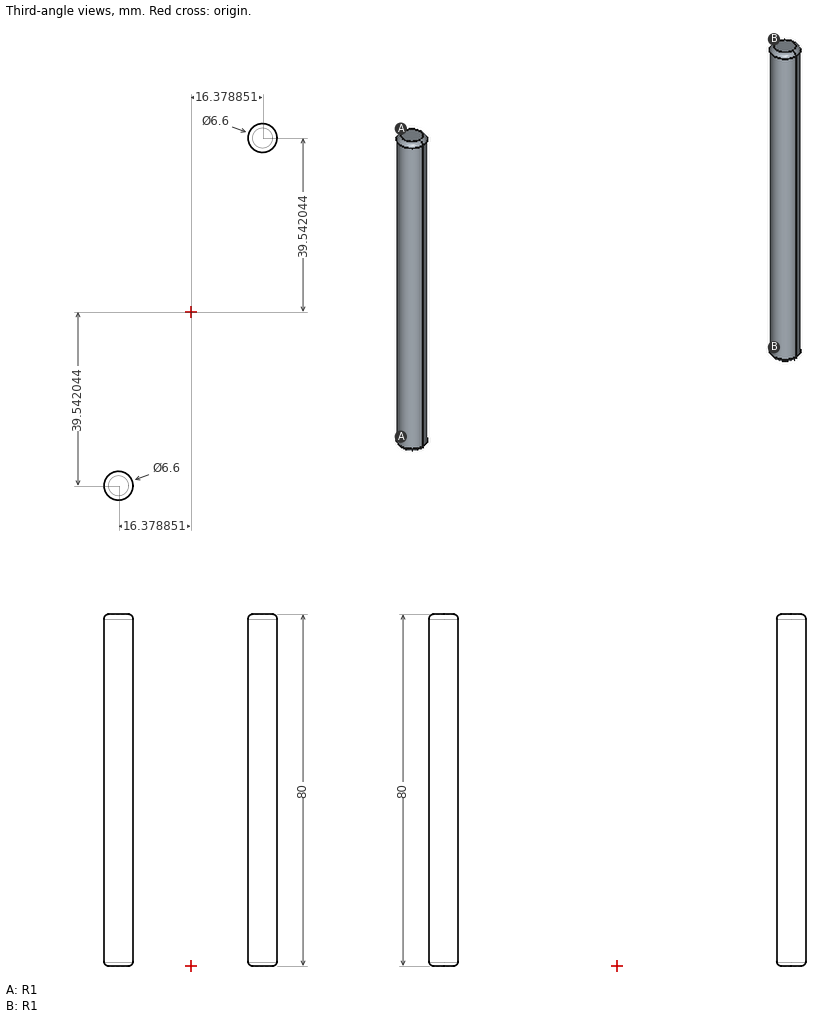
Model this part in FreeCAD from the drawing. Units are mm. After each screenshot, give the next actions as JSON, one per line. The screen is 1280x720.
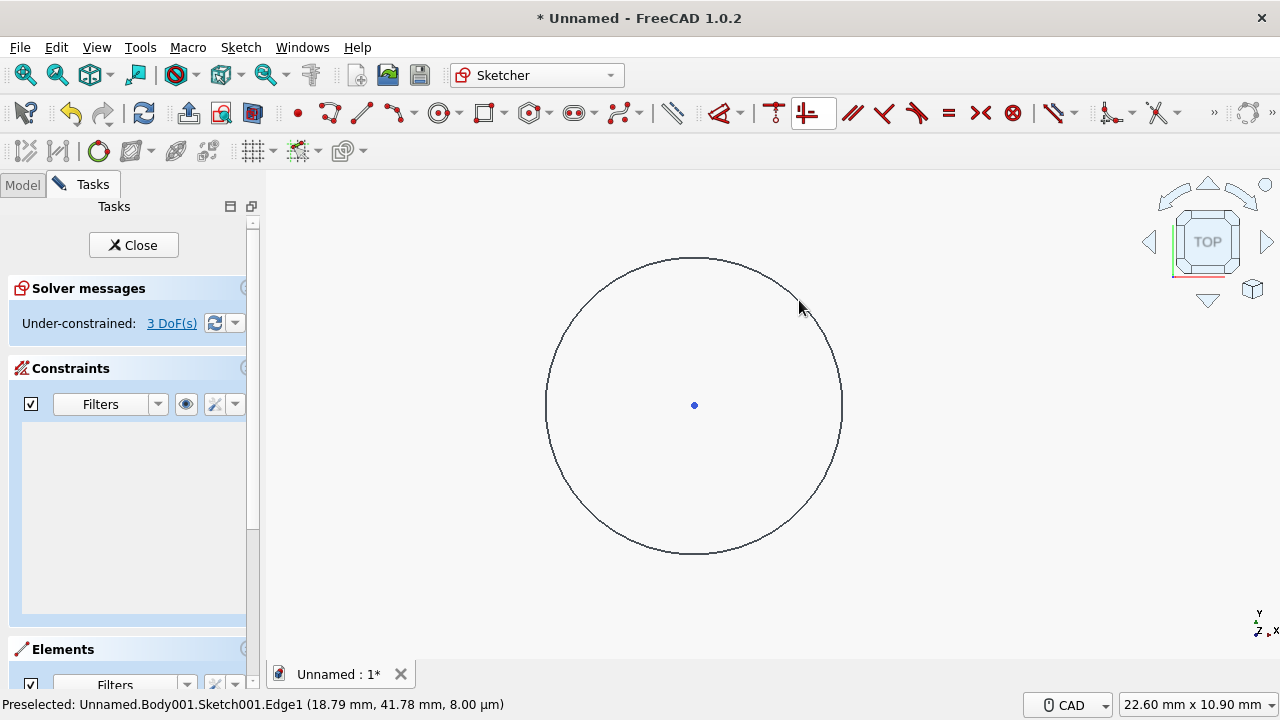
{"action": "left_click", "coordinate": [720, 114]}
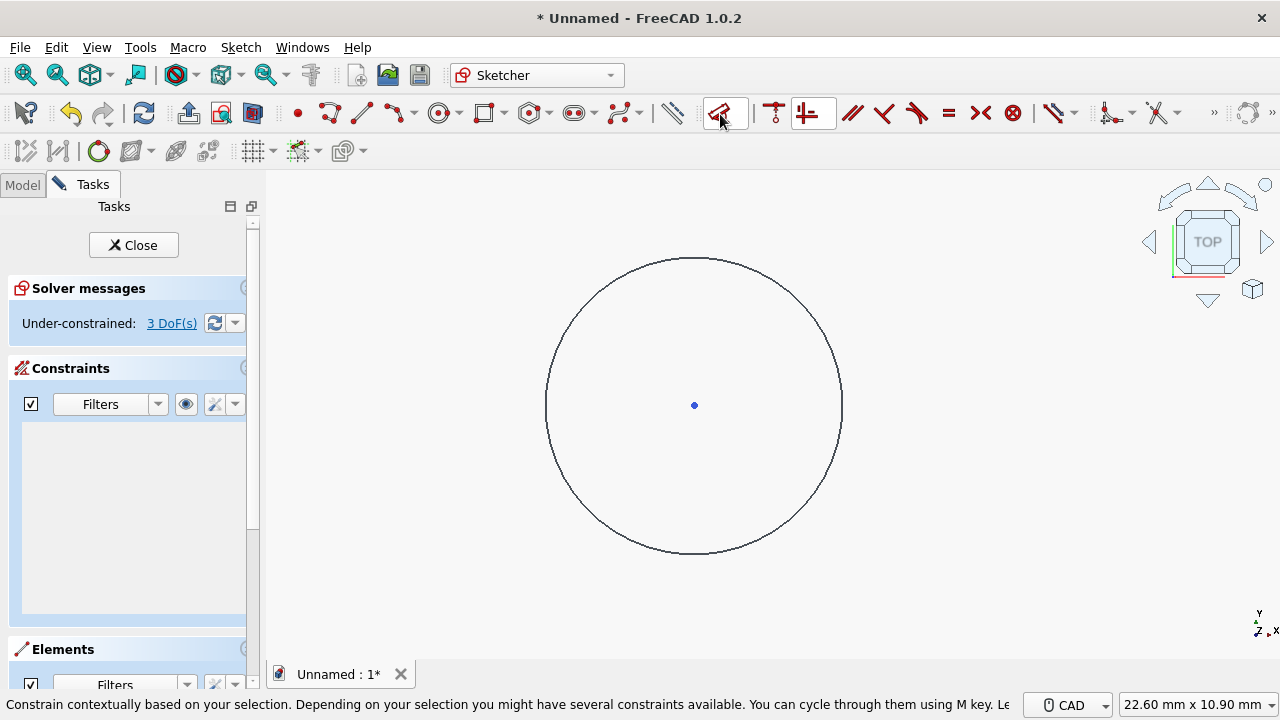
{"action": "left_click", "coordinate": [799, 301]}
{"action": "left_click", "coordinate": [822, 278]}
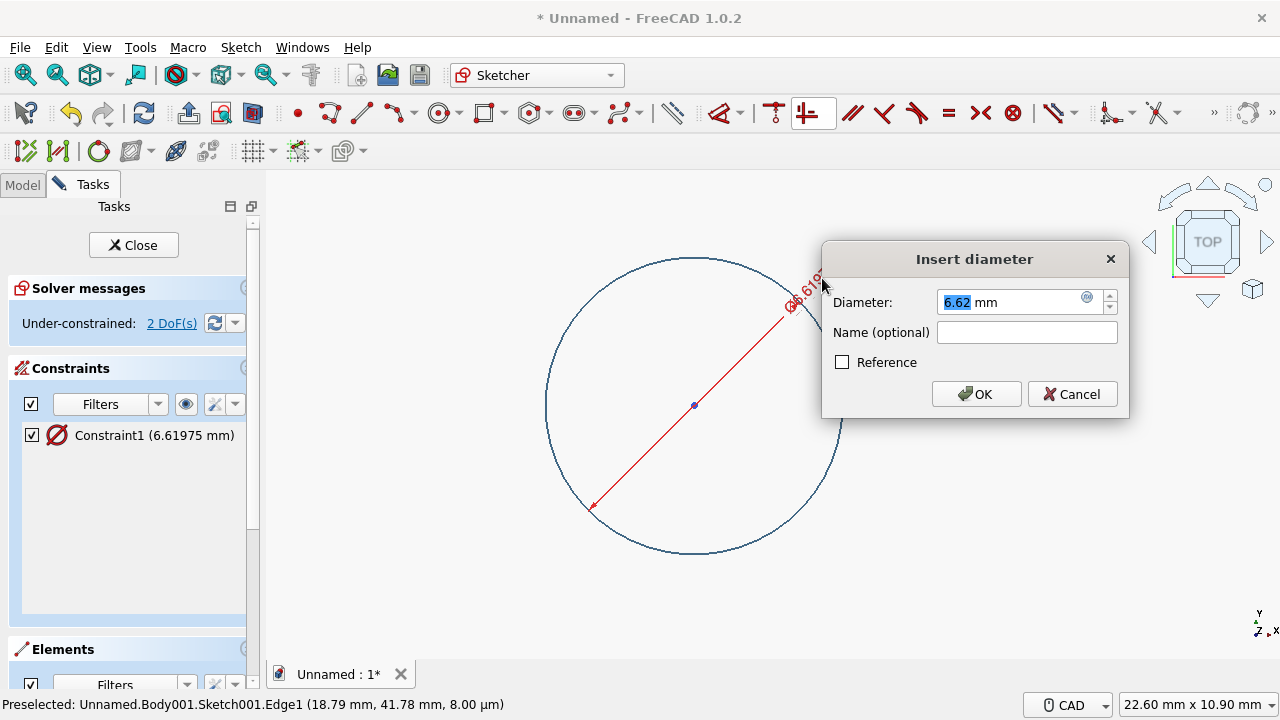
{"action": "type", "text": "6.6"}
{"action": "key", "text": "Return"}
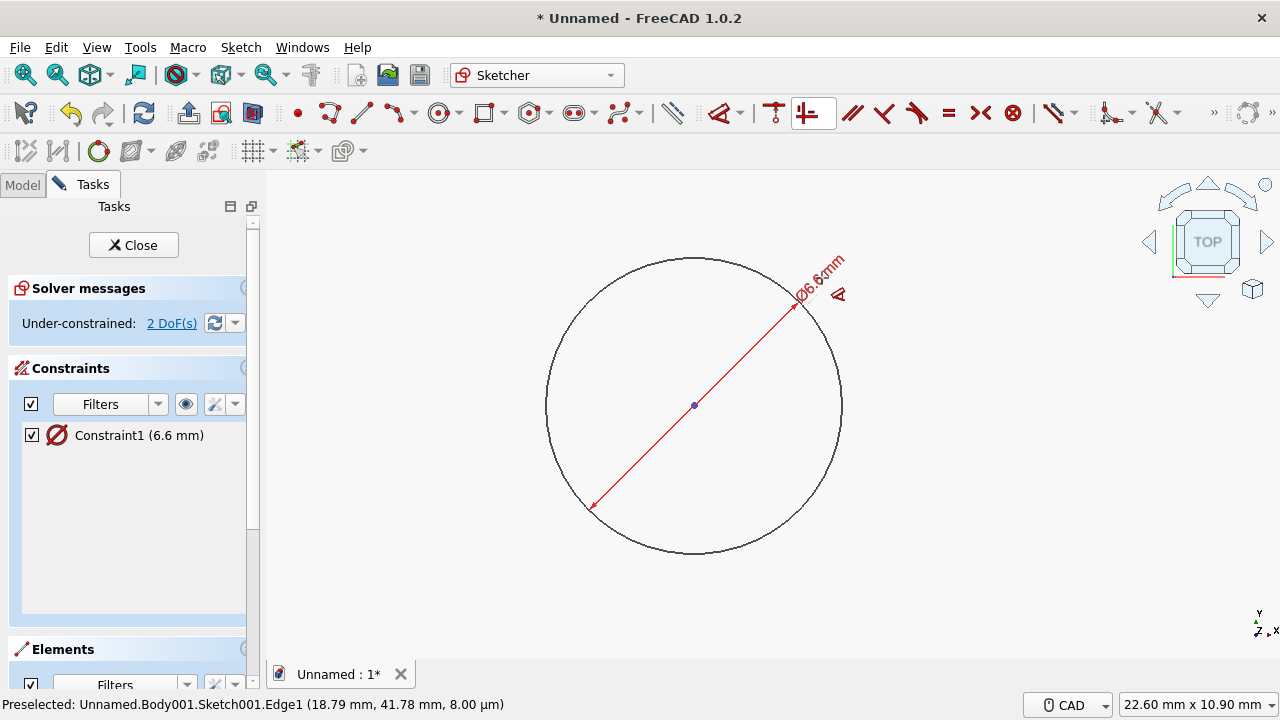
{"action": "left_click", "coordinate": [694, 406]}
{"action": "left_click", "coordinate": [494, 372]}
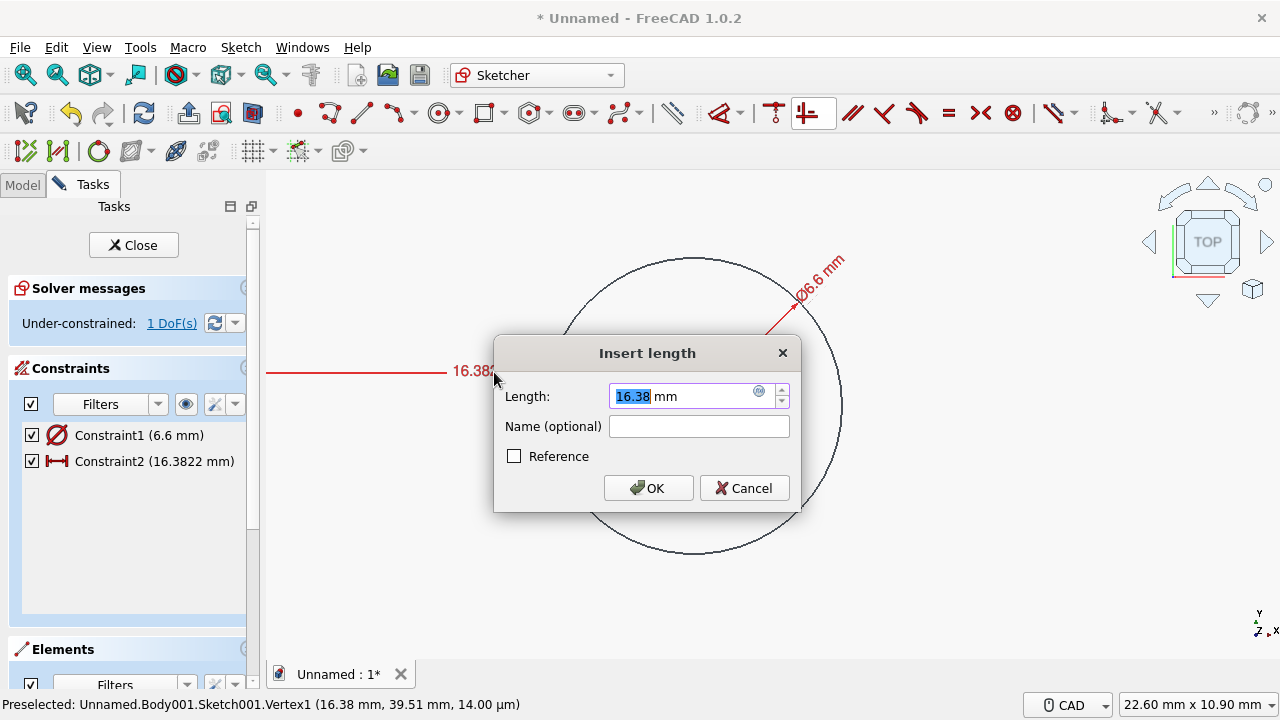
{"action": "type", "text": "16.378851"}
{"action": "key", "text": "Return"}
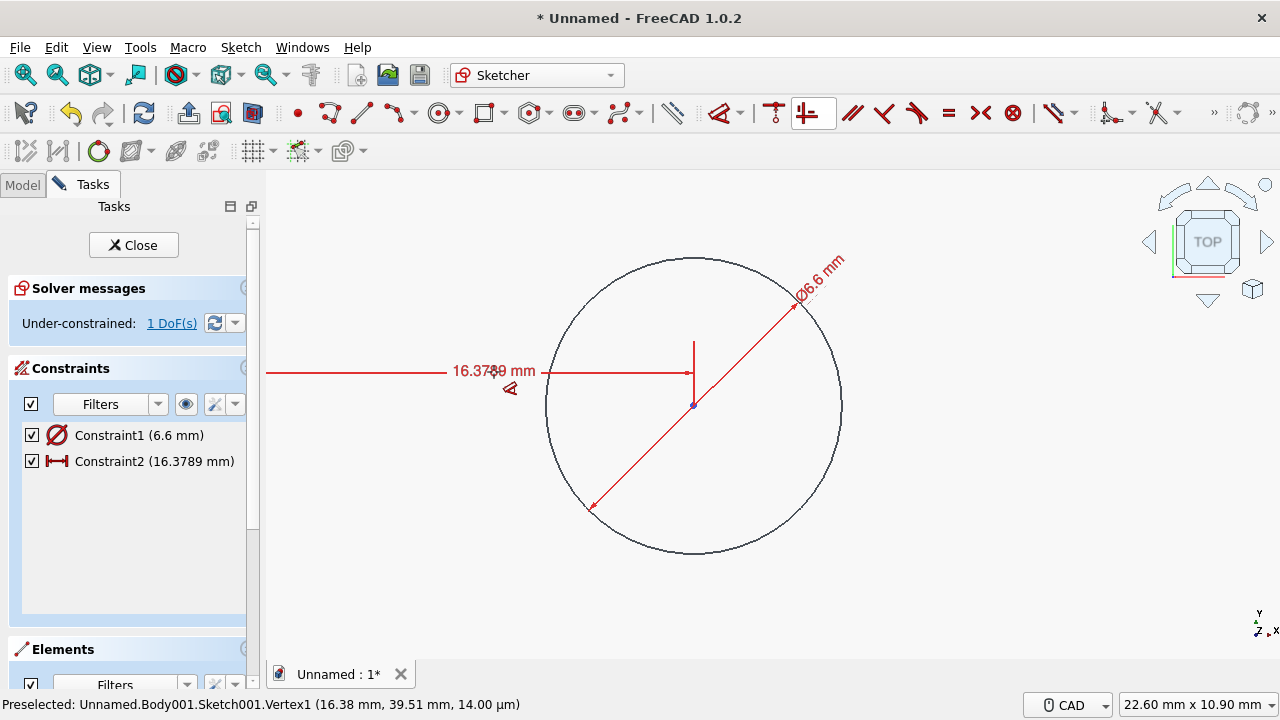
{"action": "left_click", "coordinate": [694, 406]}
{"action": "left_click", "coordinate": [728, 518]}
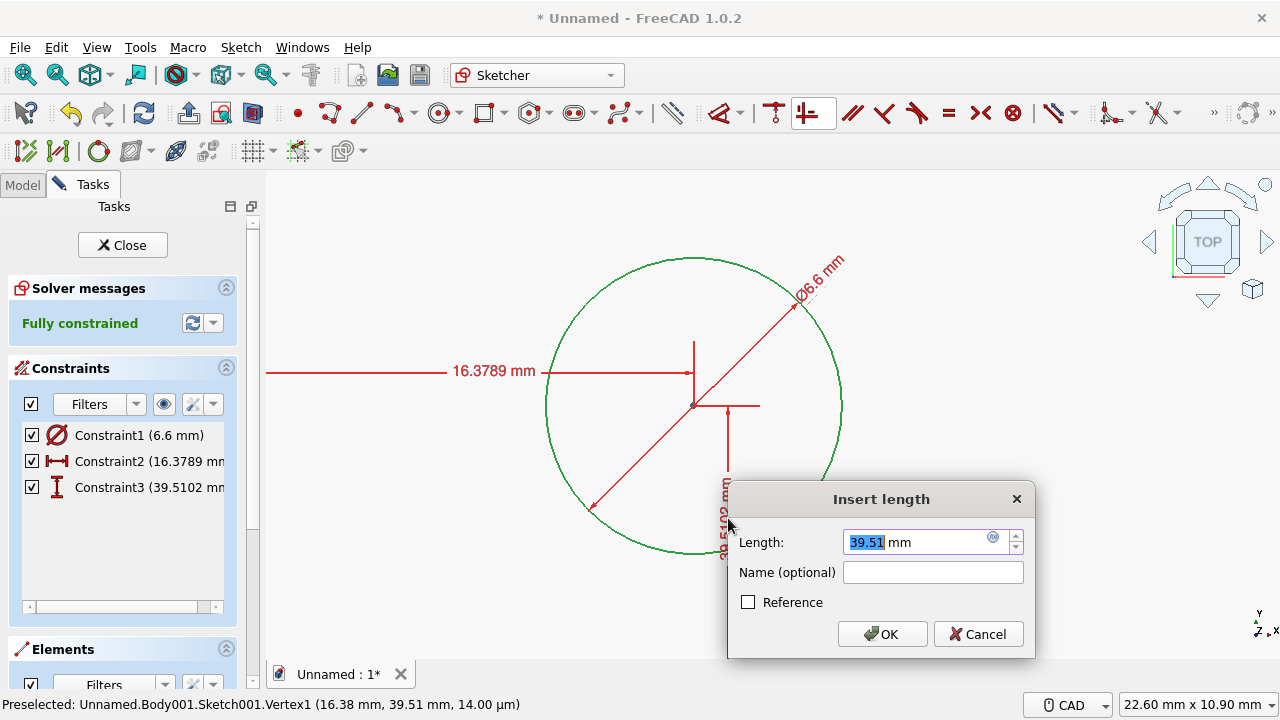
{"action": "type", "text": "39.542044"}
{"action": "key", "text": "Return"}
{"action": "key", "text": "Escape"}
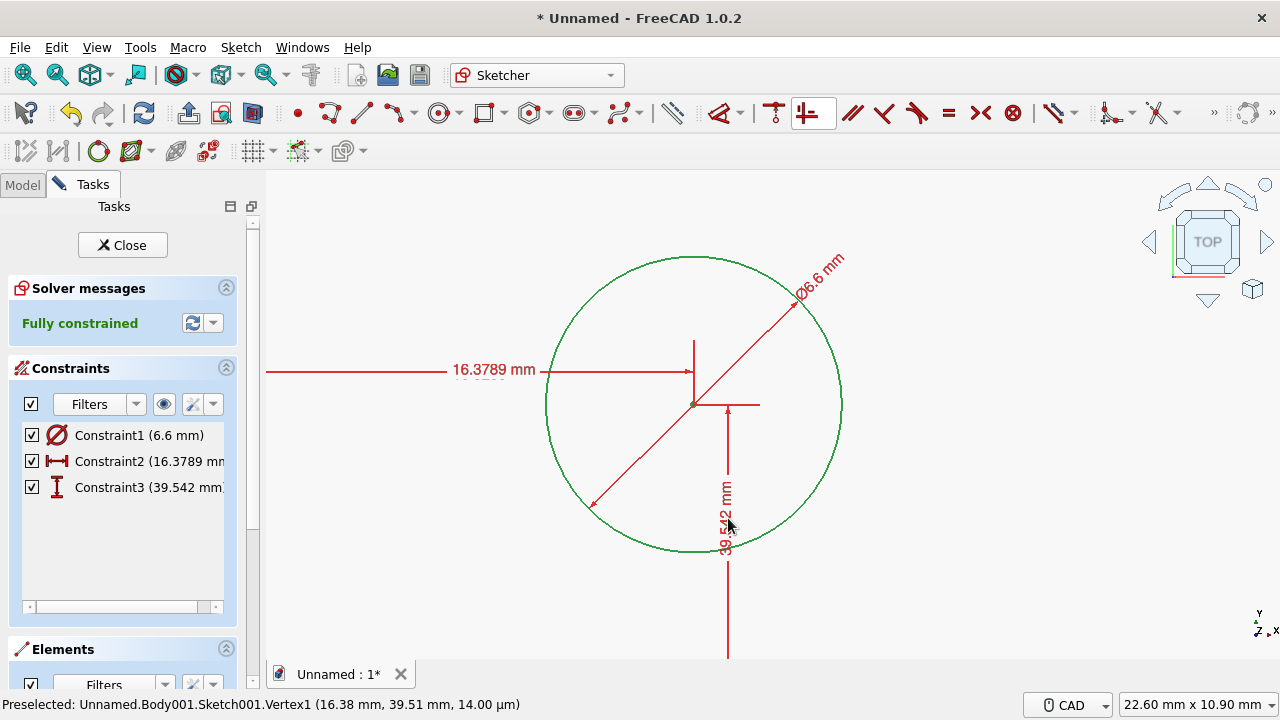
{"action": "left_click", "coordinate": [123, 245]}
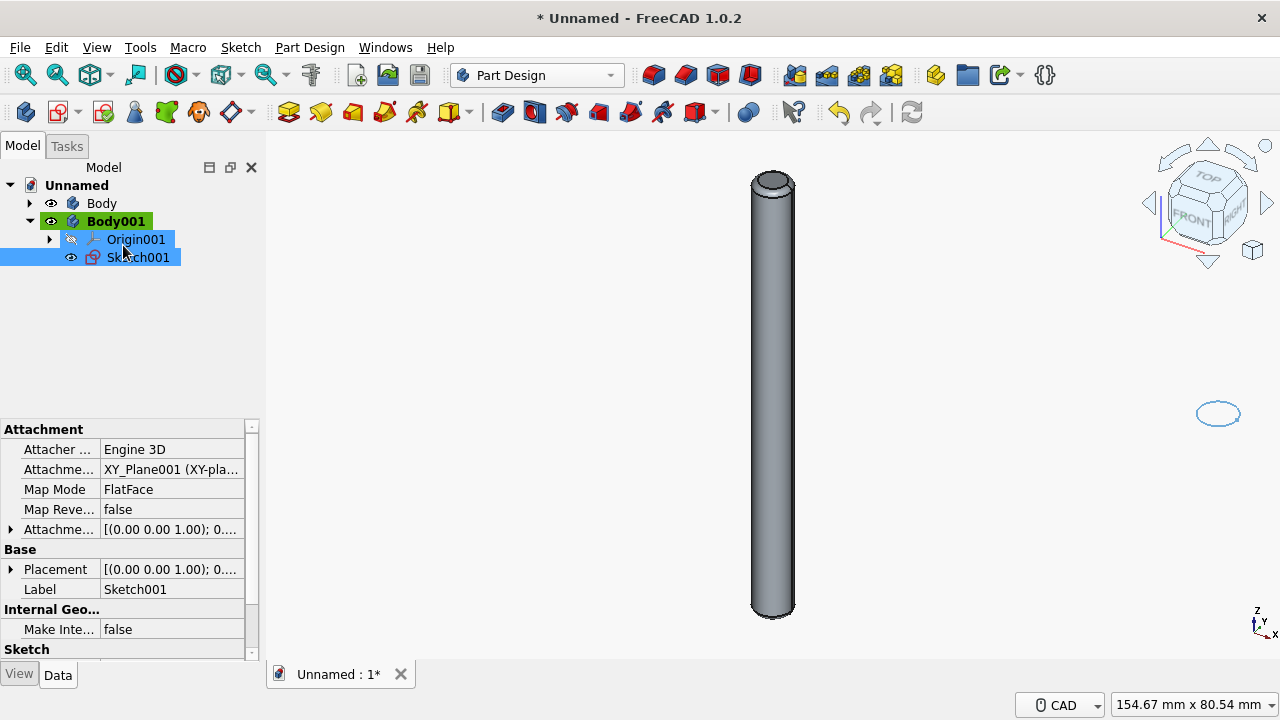
{"action": "left_click", "coordinate": [290, 112]}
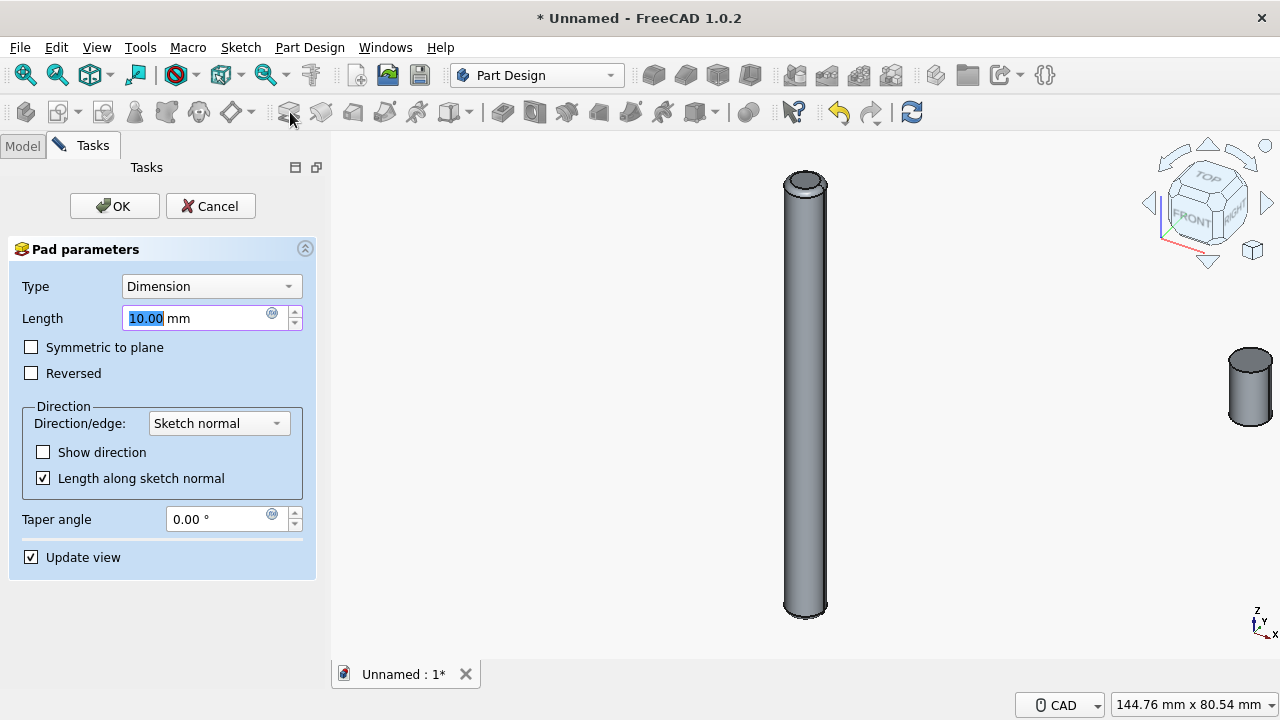
{"action": "type", "text": "80"}
{"action": "key", "text": "Tab"}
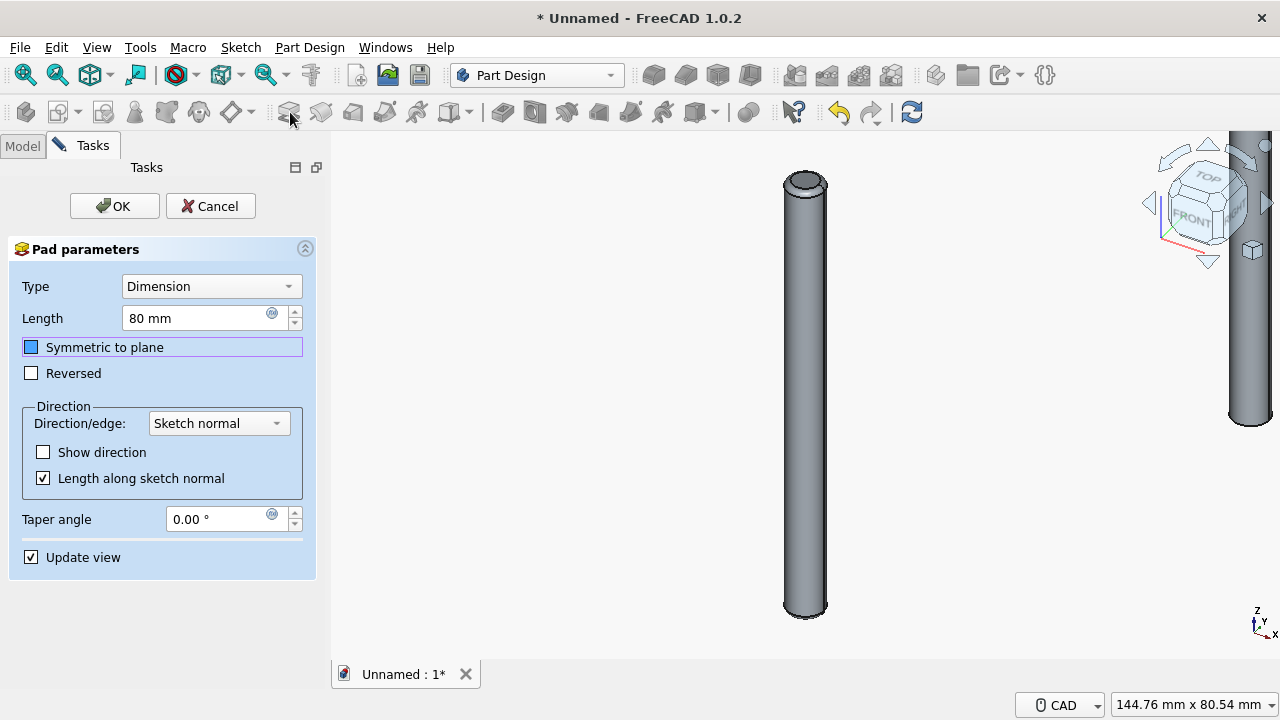
{"action": "left_click", "coordinate": [115, 206]}